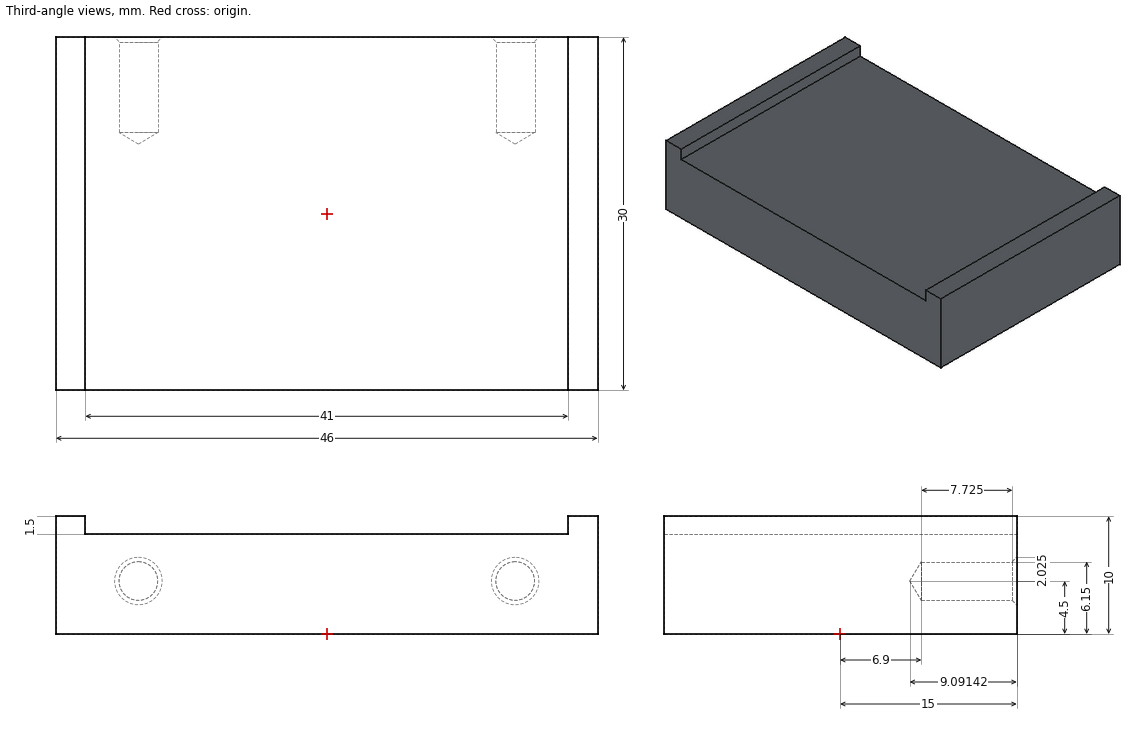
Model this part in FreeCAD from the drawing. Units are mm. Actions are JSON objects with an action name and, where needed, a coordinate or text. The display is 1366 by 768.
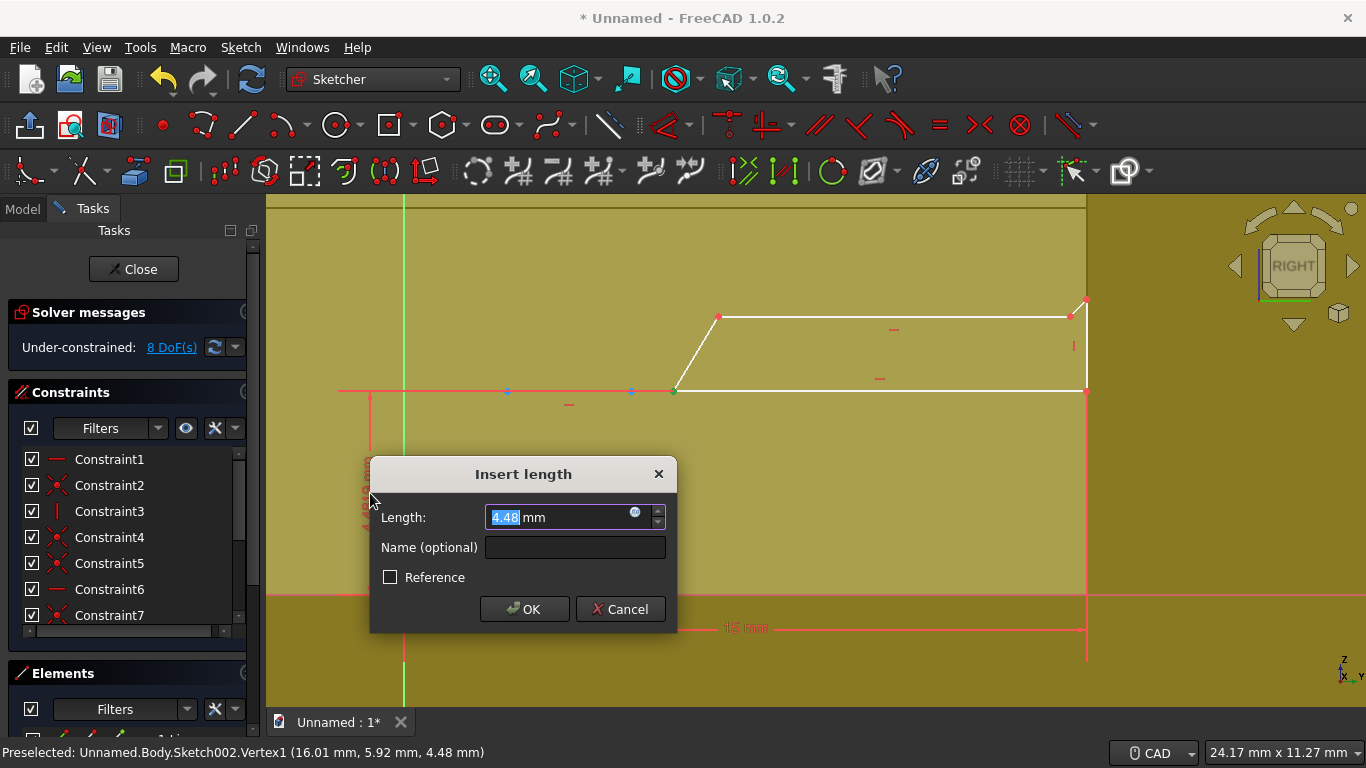
{"action": "type", "text": "4.5"}
{"action": "key", "text": "Return"}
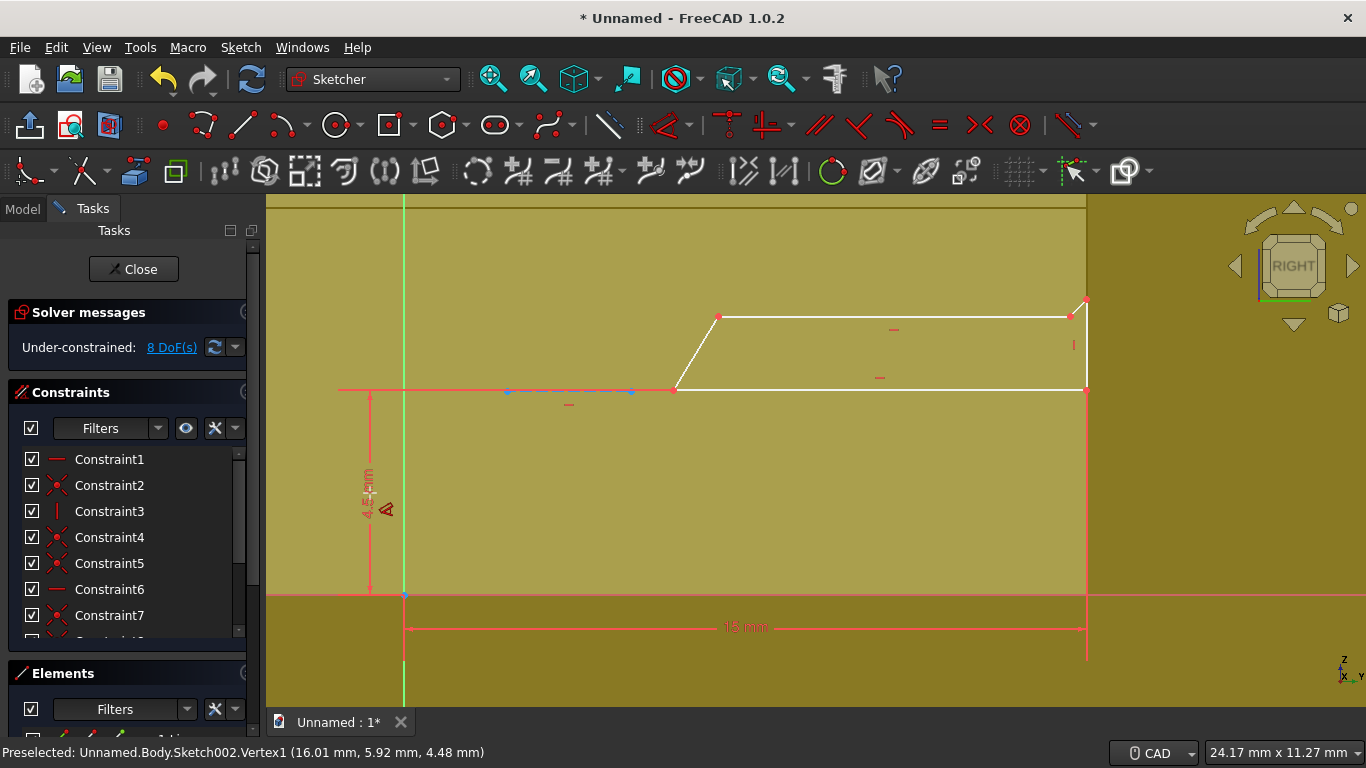
{"action": "left_click", "coordinate": [718, 317]}
{"action": "left_click", "coordinate": [561, 629]}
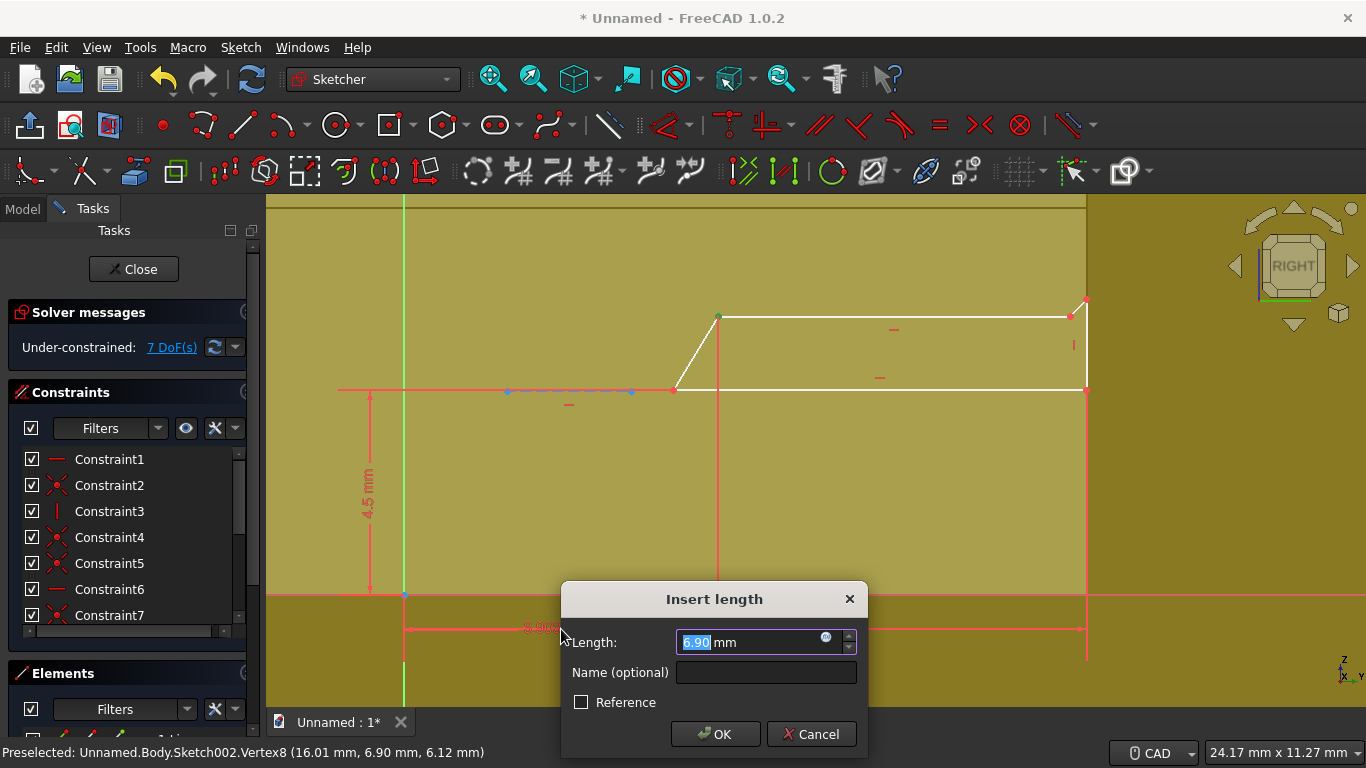
{"action": "type", "text": "6.9"}
{"action": "key", "text": "Return"}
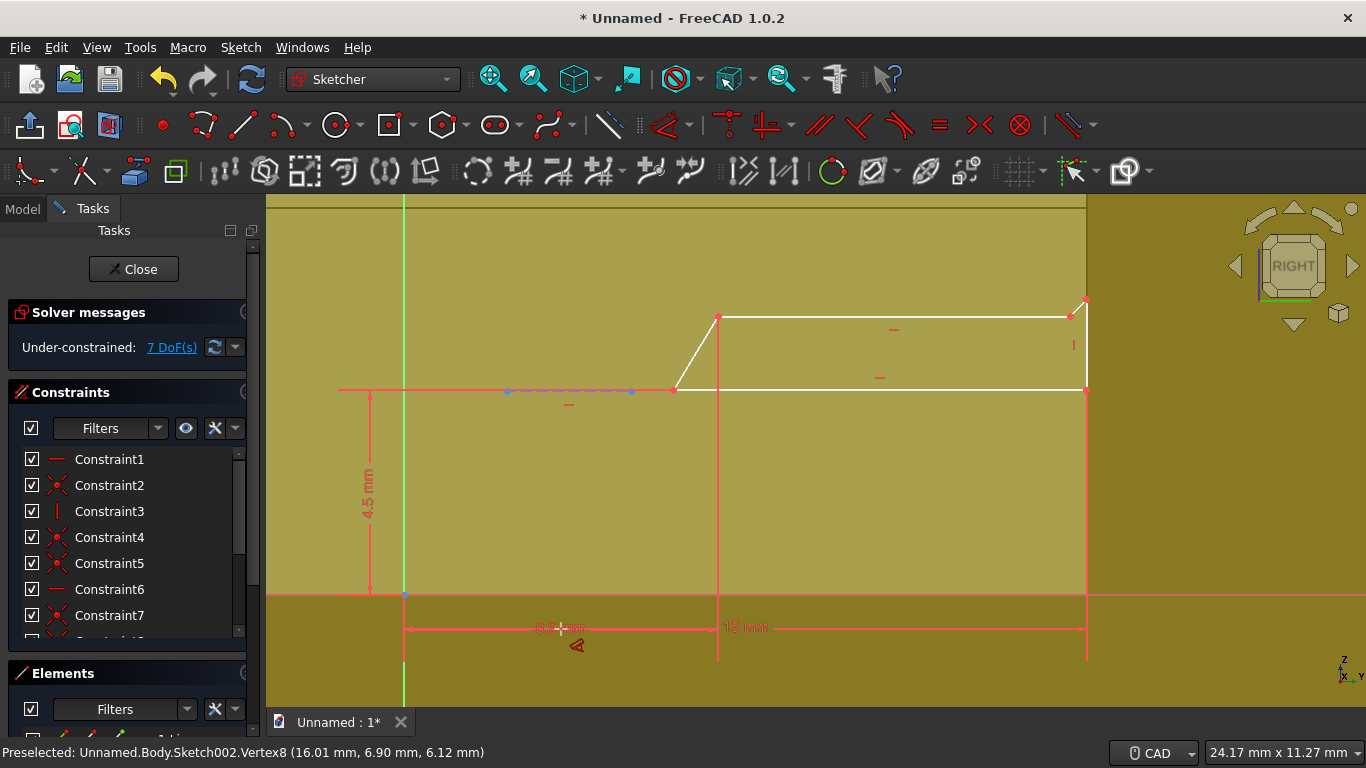
{"action": "left_click", "coordinate": [632, 391]}
{"action": "left_click", "coordinate": [370, 446]}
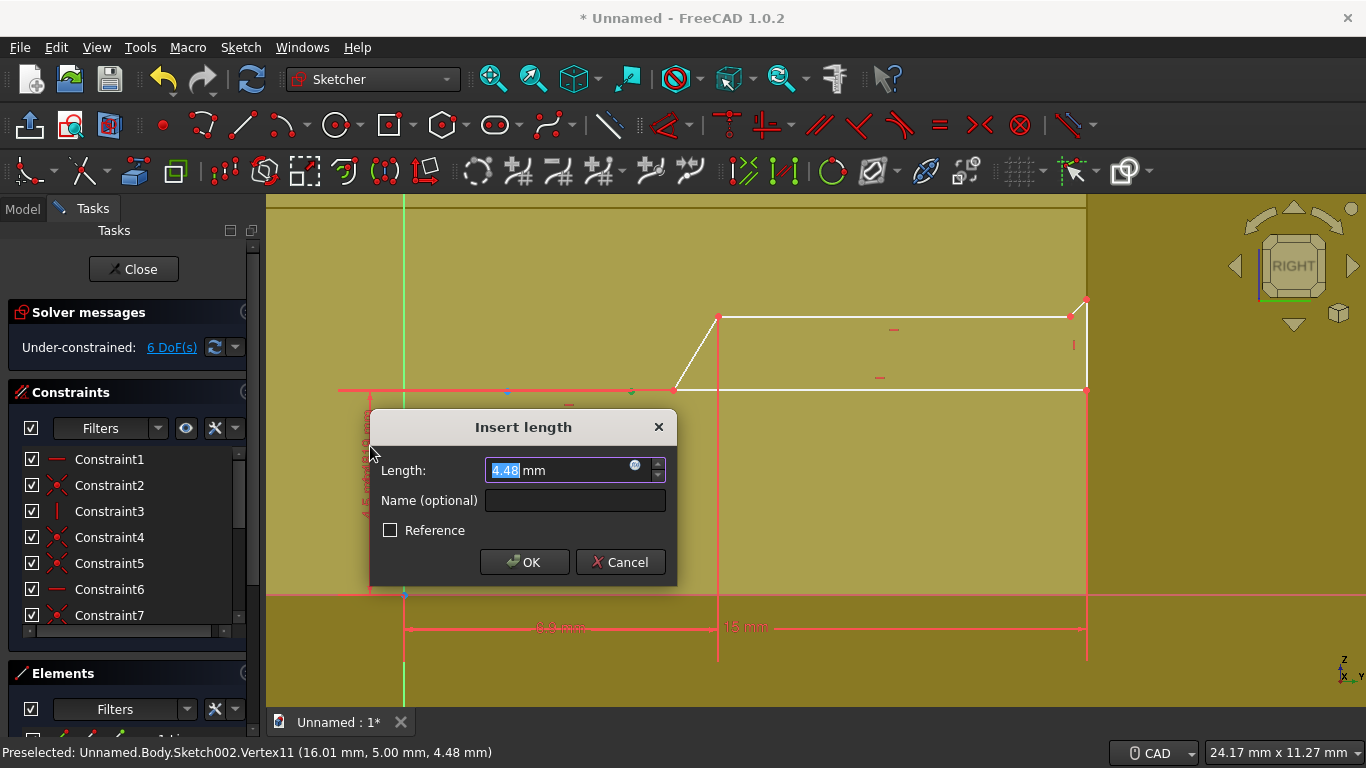
{"action": "type", "text": "4.5"}
{"action": "key", "text": "Return"}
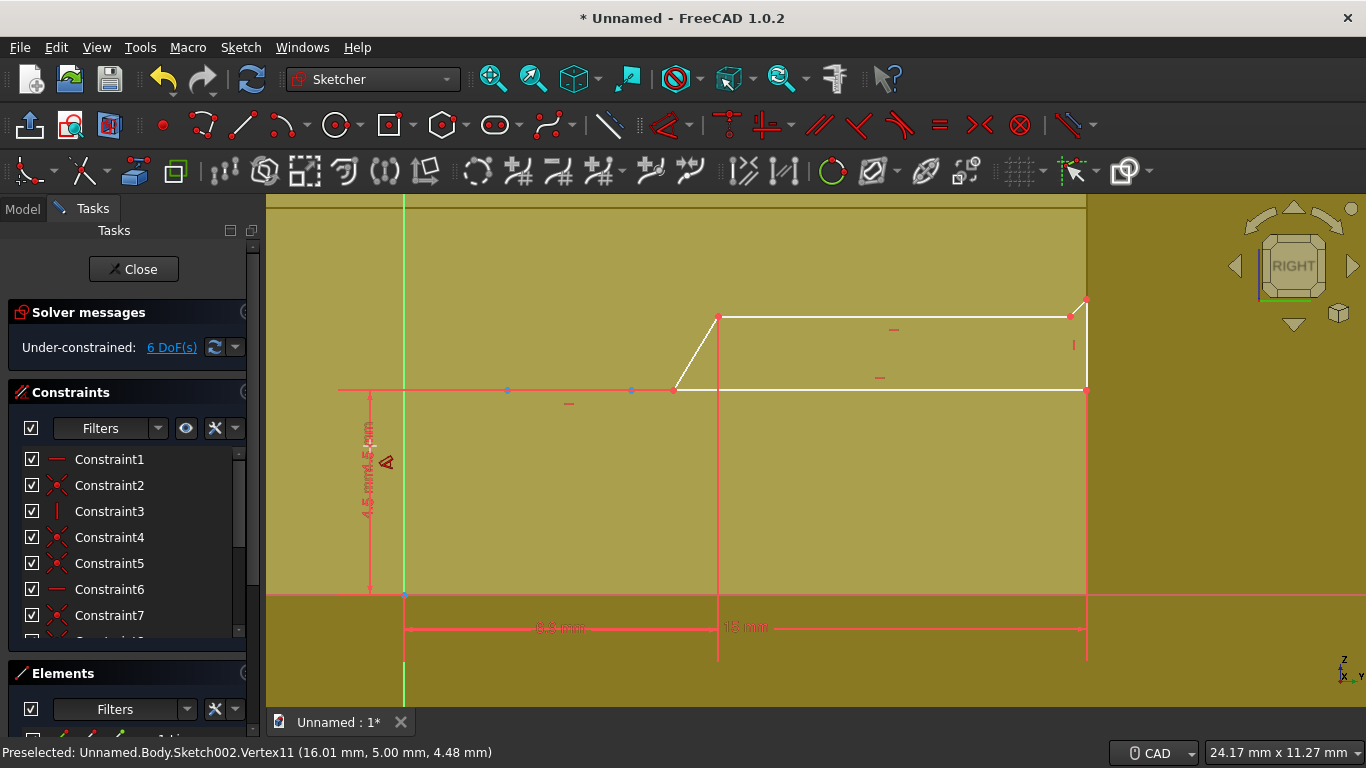
{"action": "left_click", "coordinate": [1087, 363]}
{"action": "left_click", "coordinate": [1121, 345]}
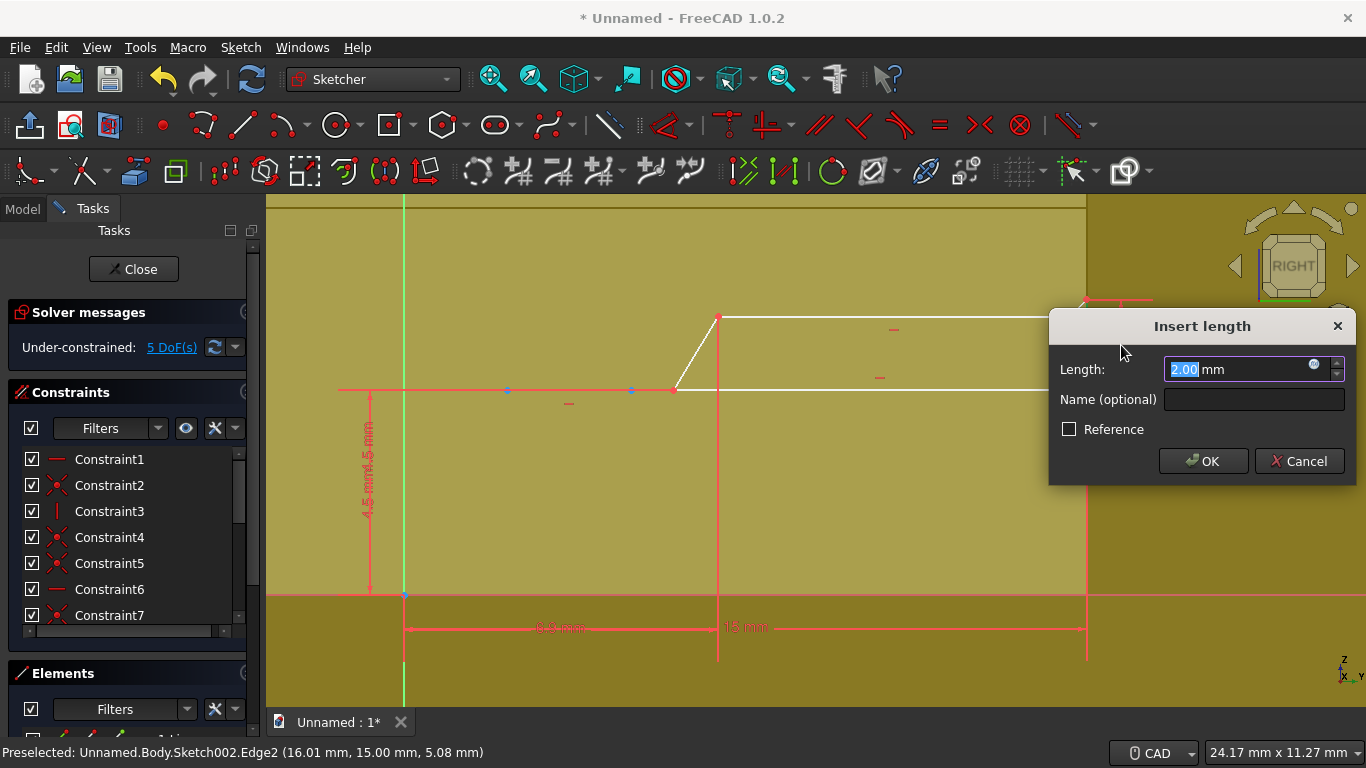
{"action": "type", "text": "2.025"}
{"action": "key", "text": "Return"}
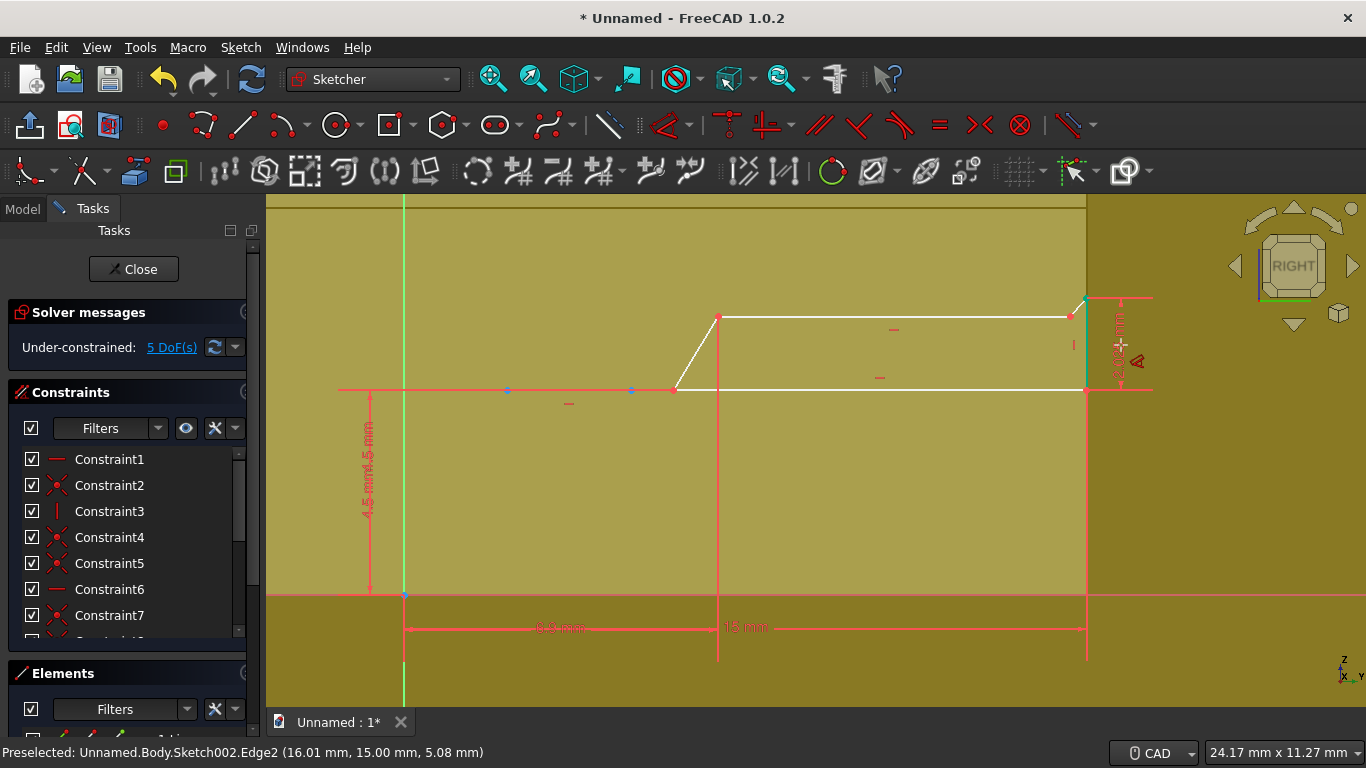
{"action": "left_click", "coordinate": [964, 317]}
{"action": "left_click", "coordinate": [894, 283]}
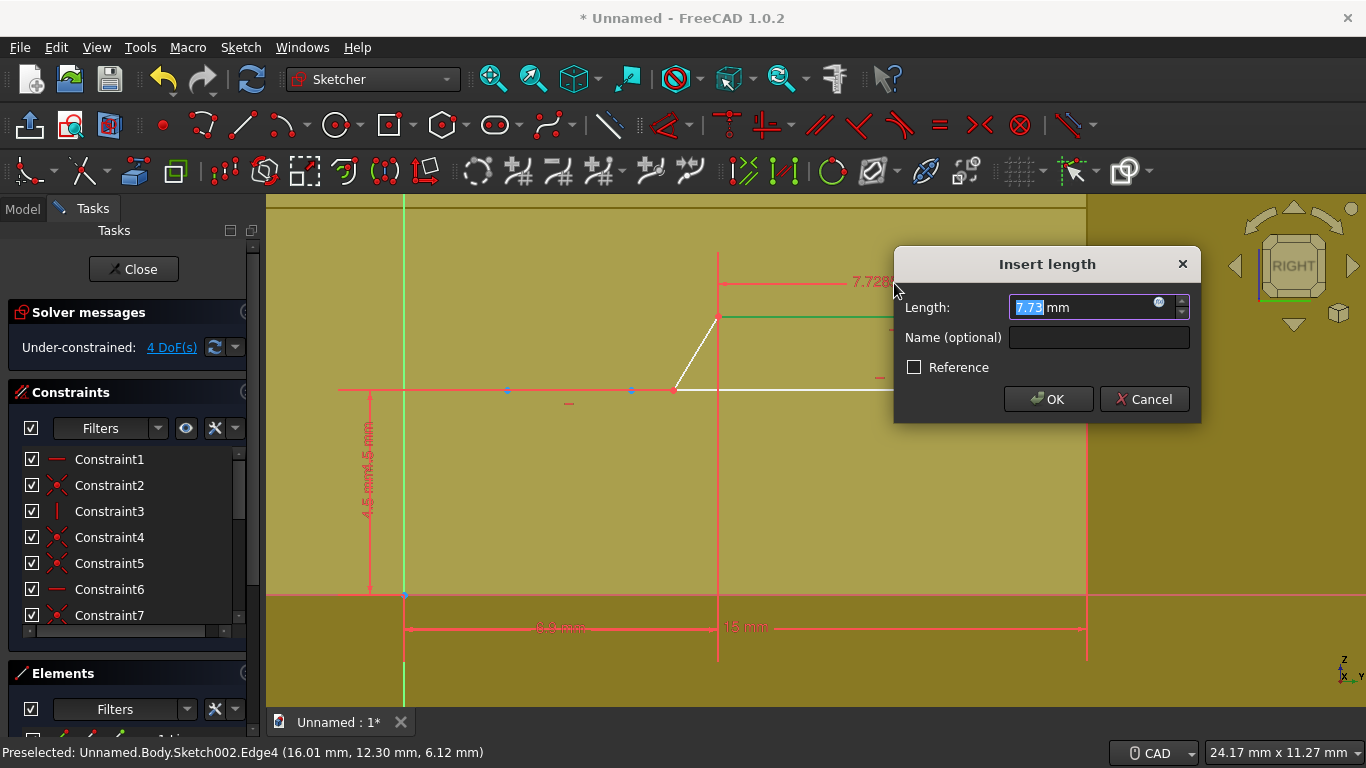
{"action": "type", "text": "7.725"}
{"action": "key", "text": "Return"}